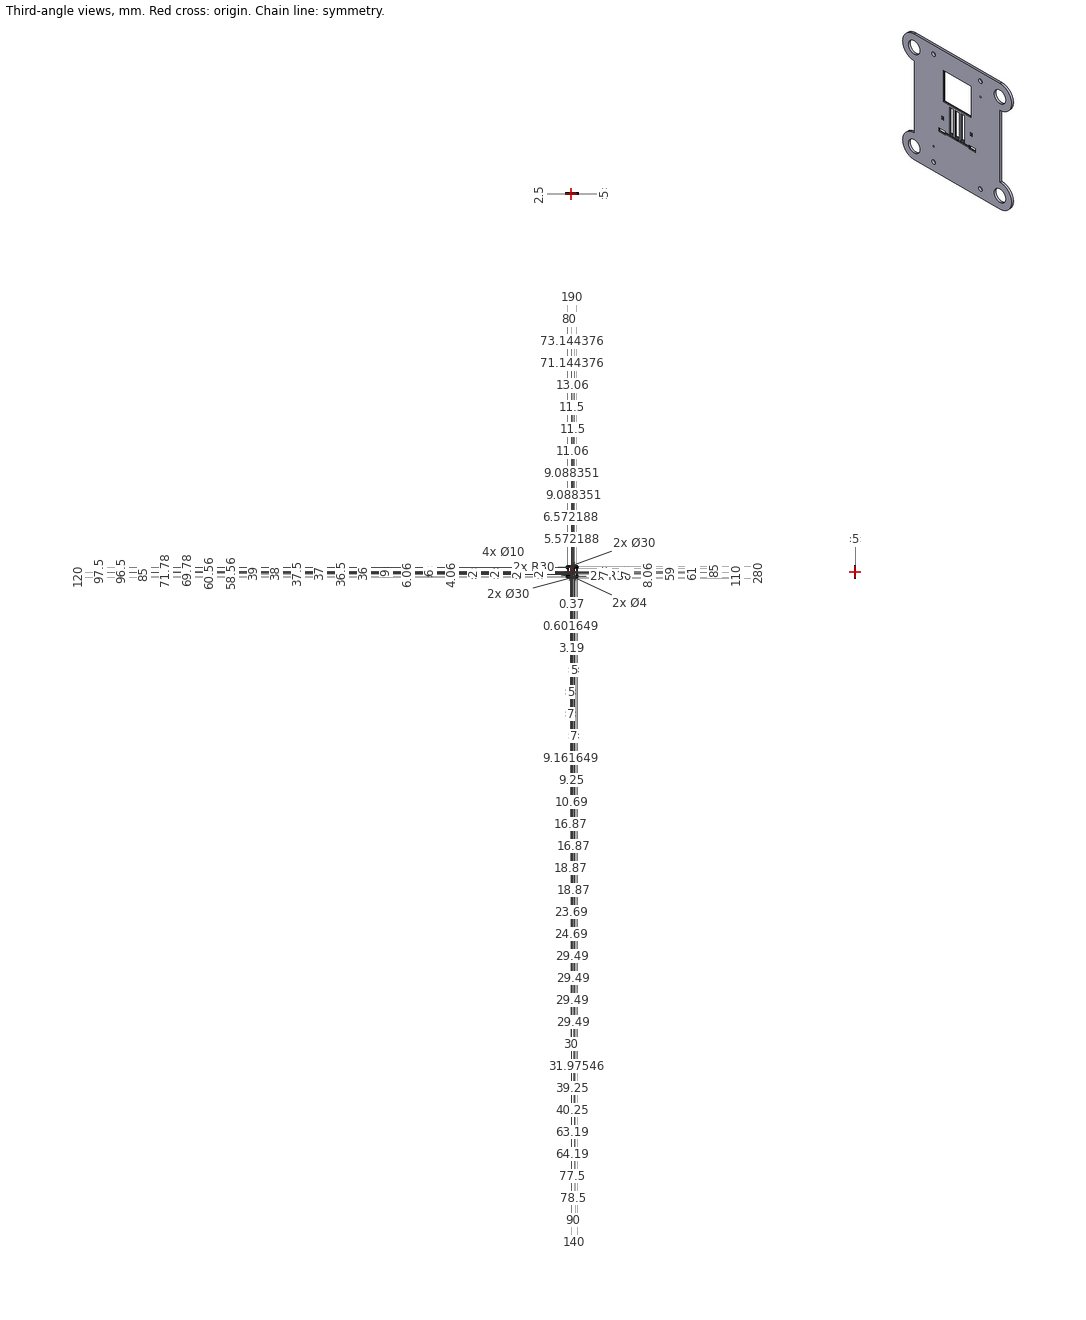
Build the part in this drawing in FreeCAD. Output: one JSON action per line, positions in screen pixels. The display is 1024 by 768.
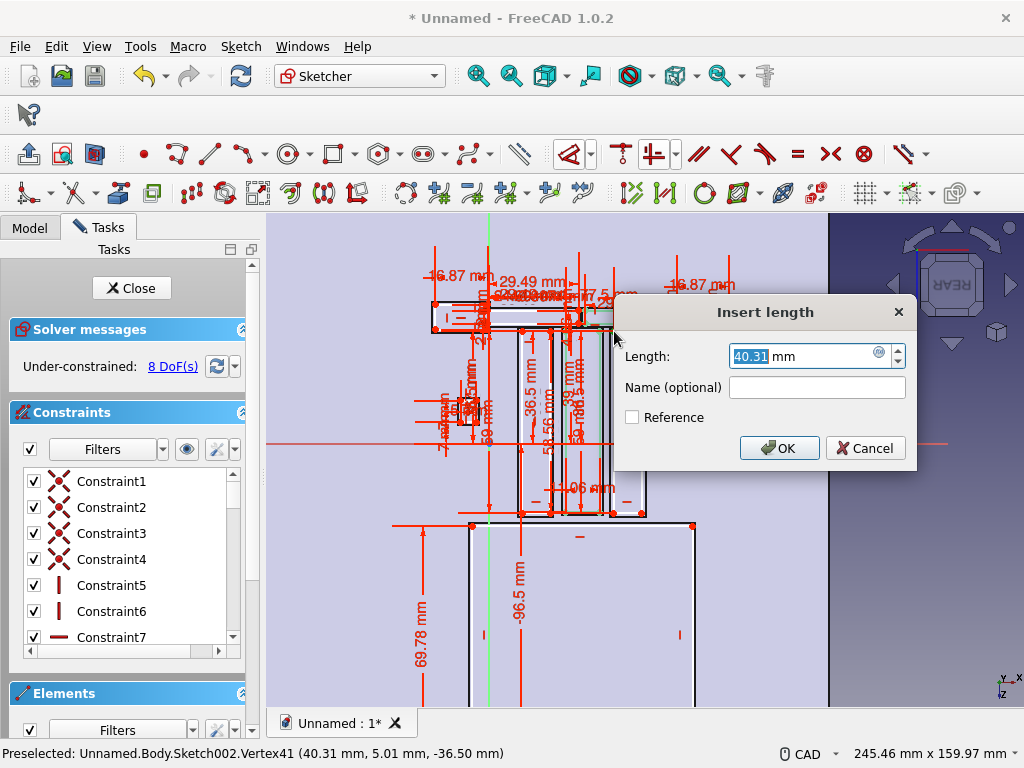
{"action": "type", "text": "40.25"}
{"action": "key", "text": "Return"}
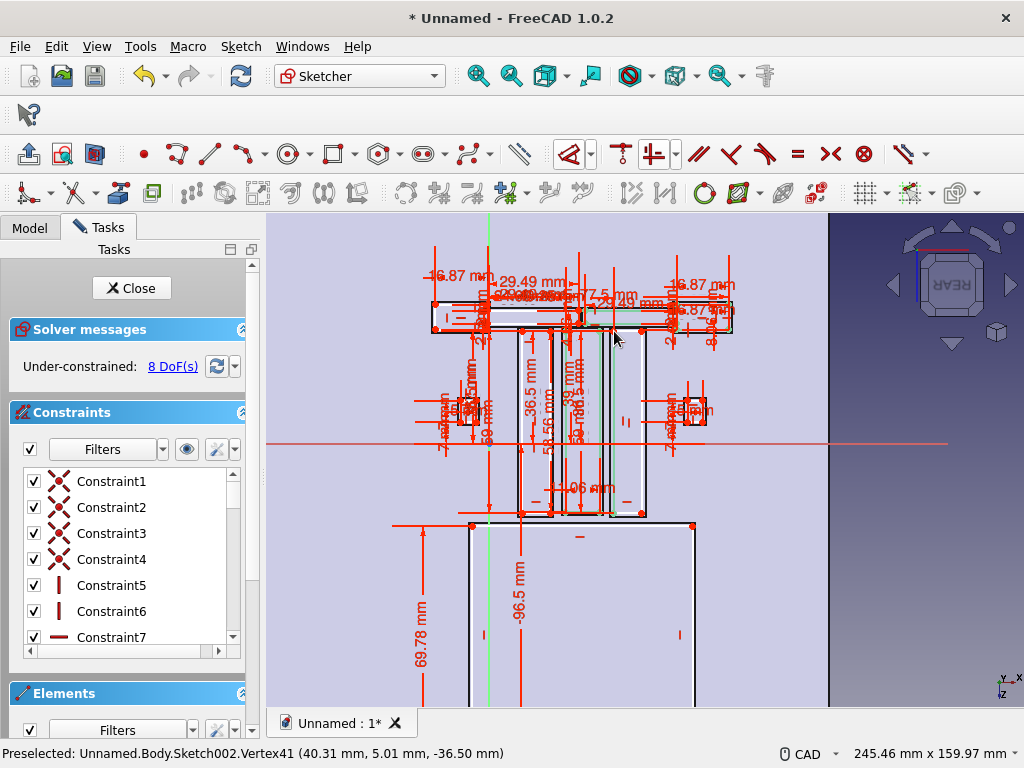
{"action": "left_click", "coordinate": [688, 401]}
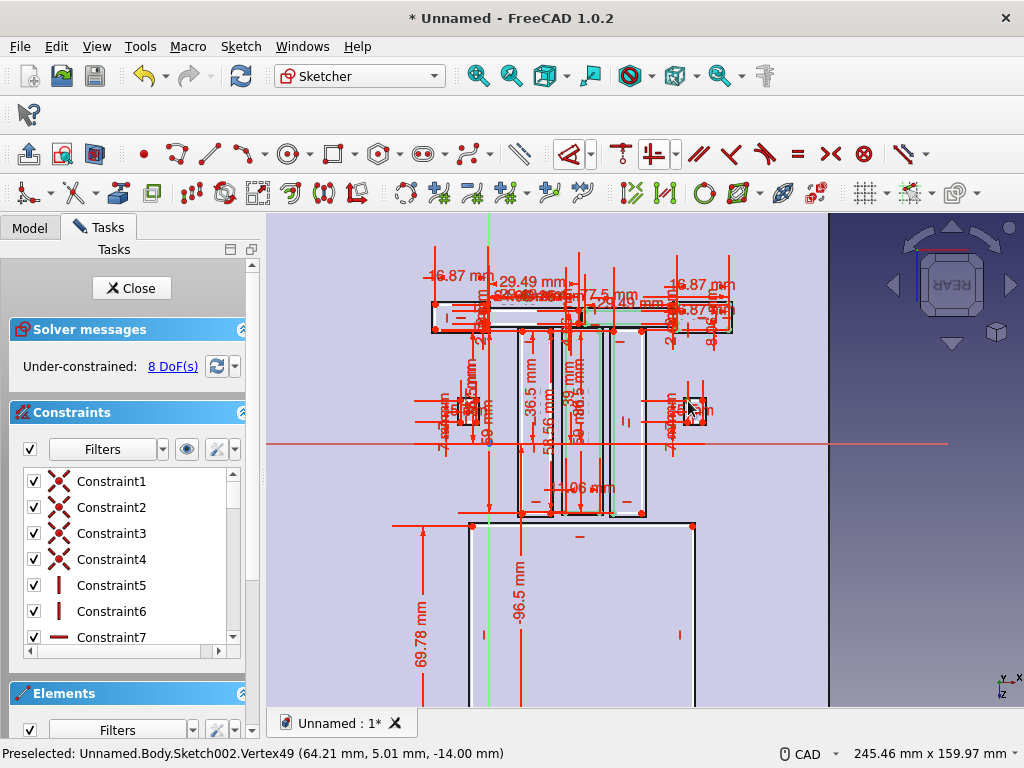
{"action": "key", "text": "l"}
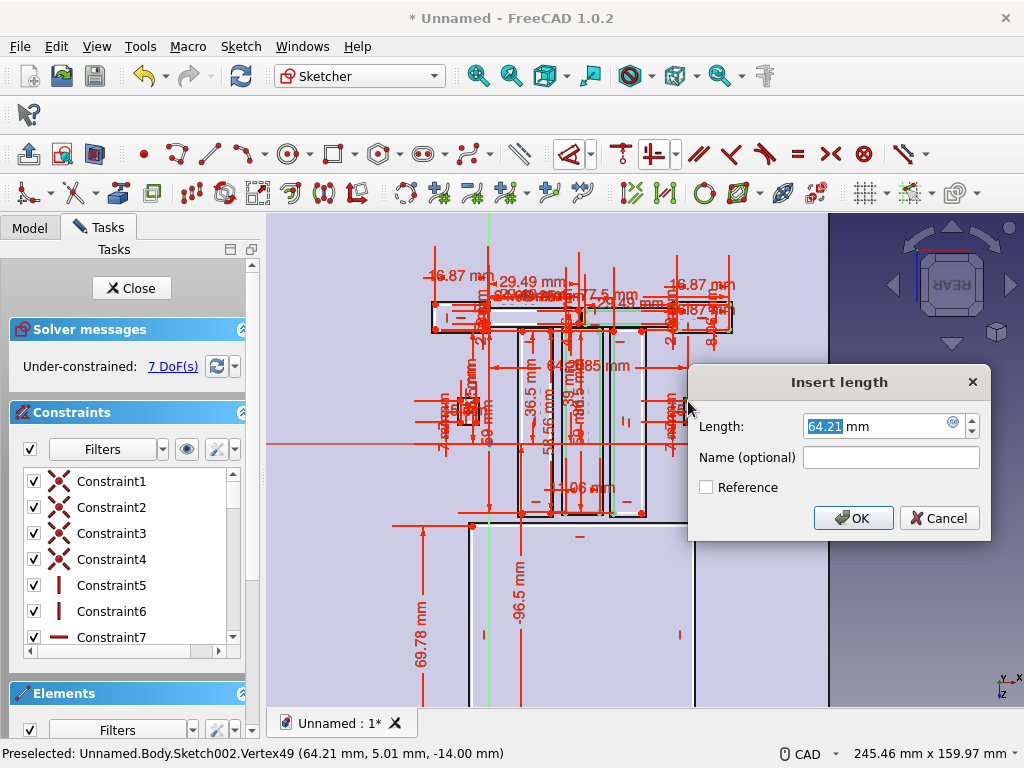
{"action": "type", "text": "64.19"}
{"action": "key", "text": "Return"}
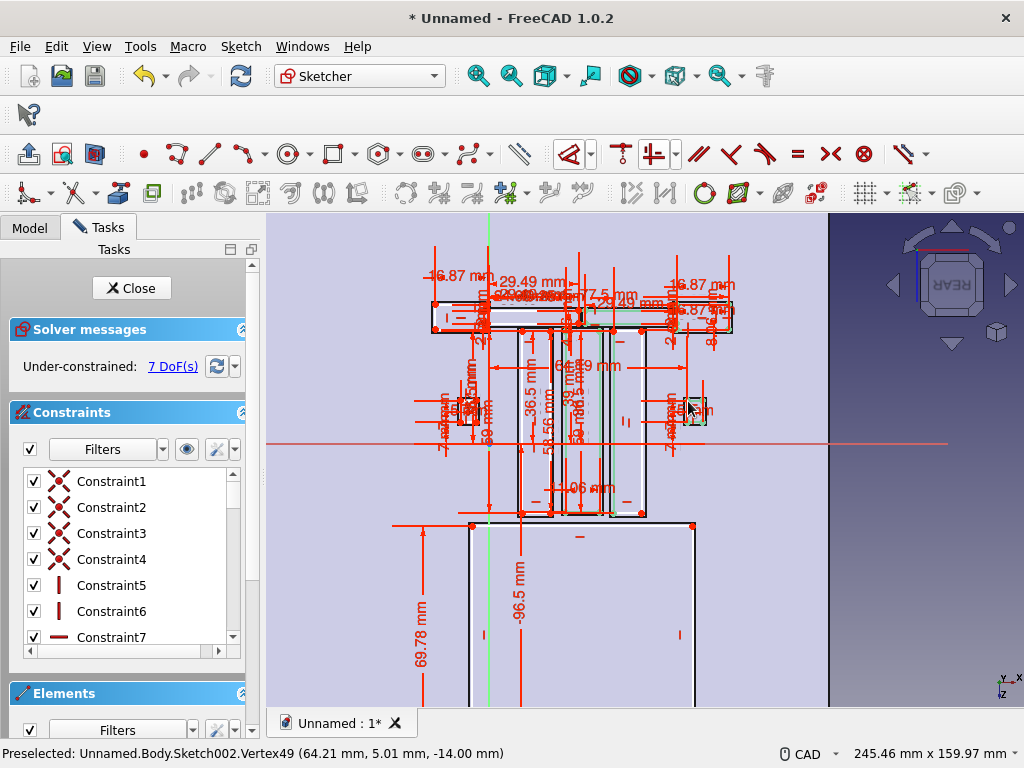
{"action": "left_click", "coordinate": [522, 331]}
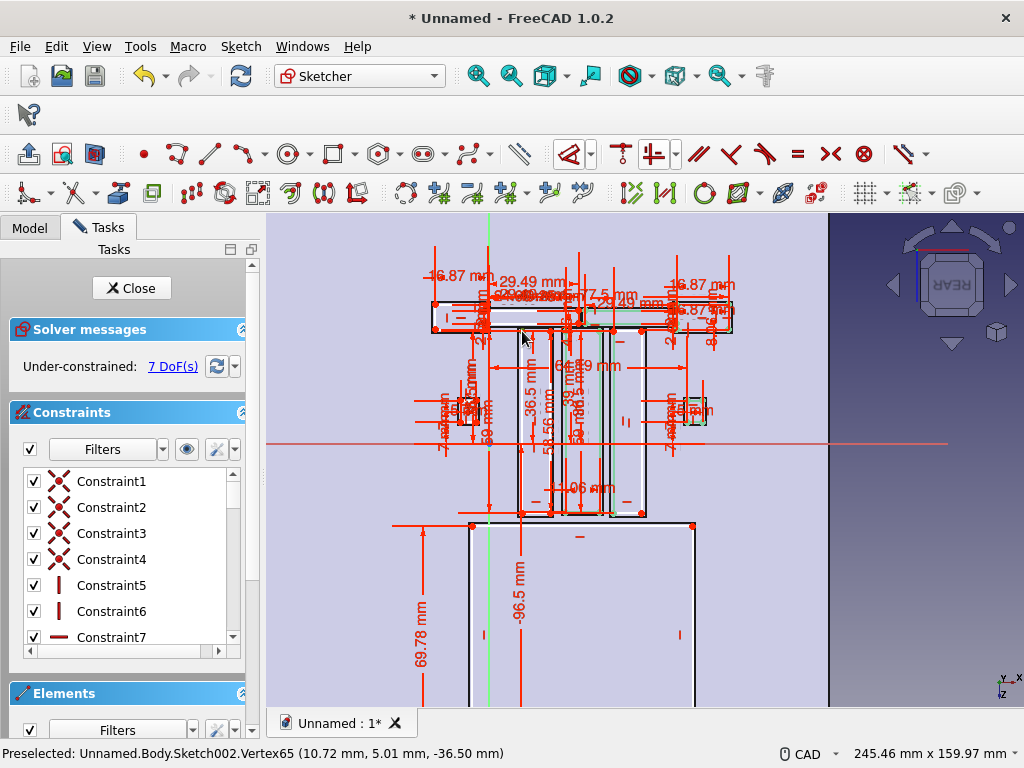
{"action": "key", "text": "l"}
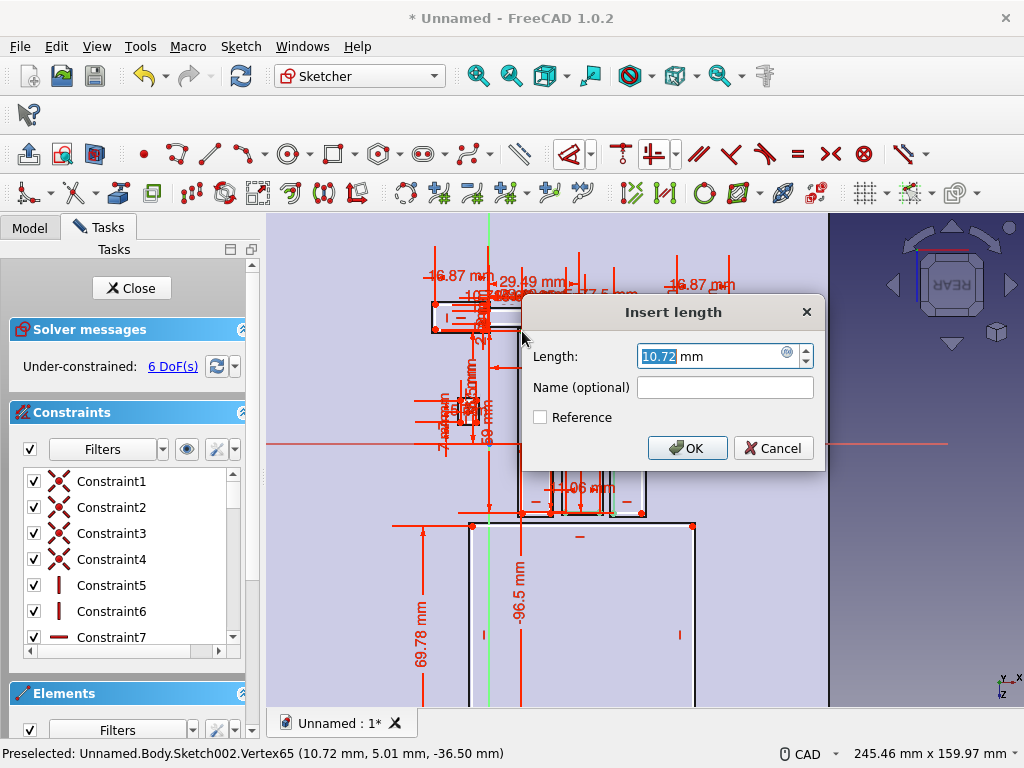
{"action": "type", "text": "10.69"}
{"action": "key", "text": "Return"}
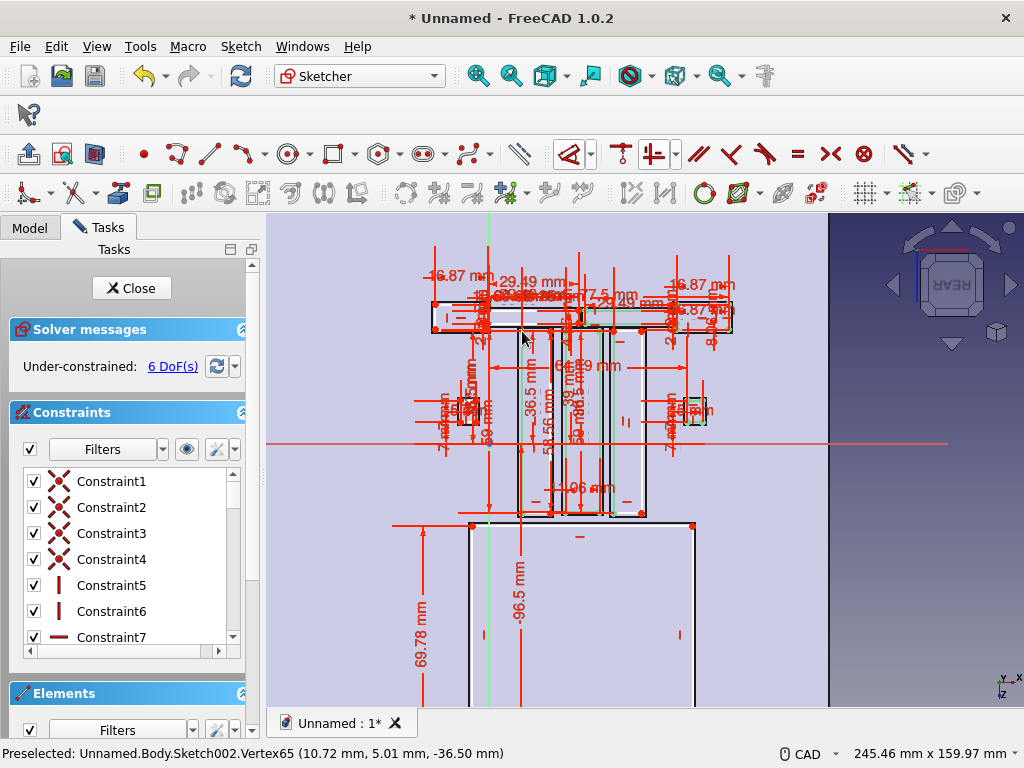
{"action": "scroll", "coordinate": [625, 513], "scroll_direction": "up", "scroll_amount": 2}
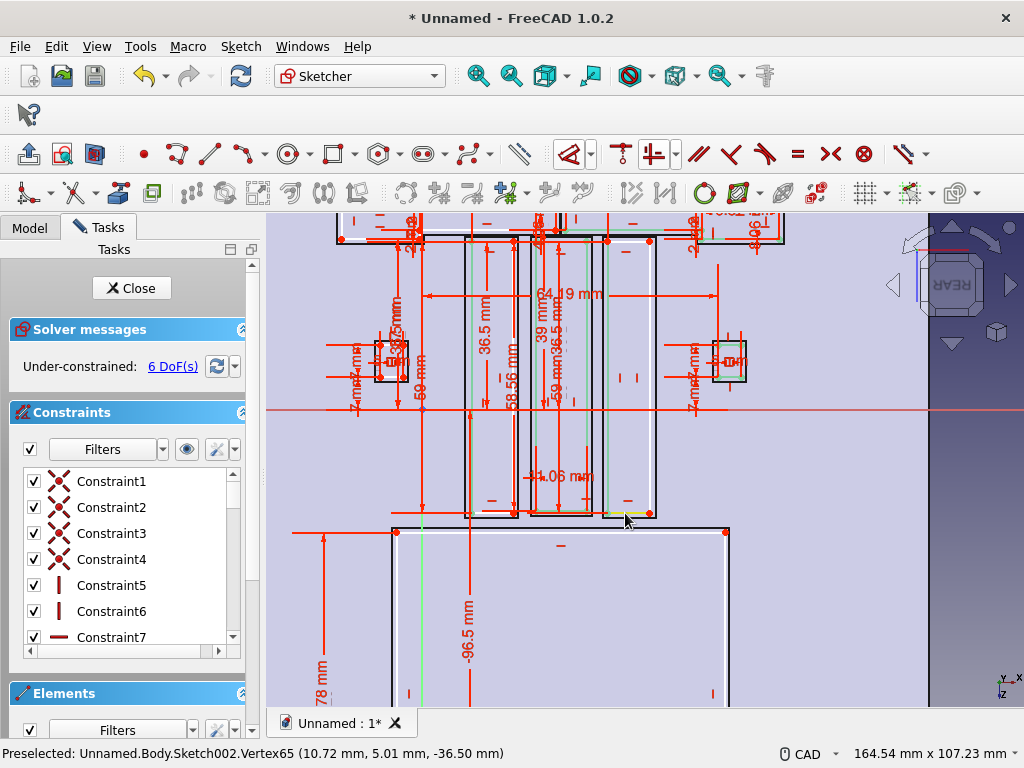
{"action": "left_click", "coordinate": [625, 513]}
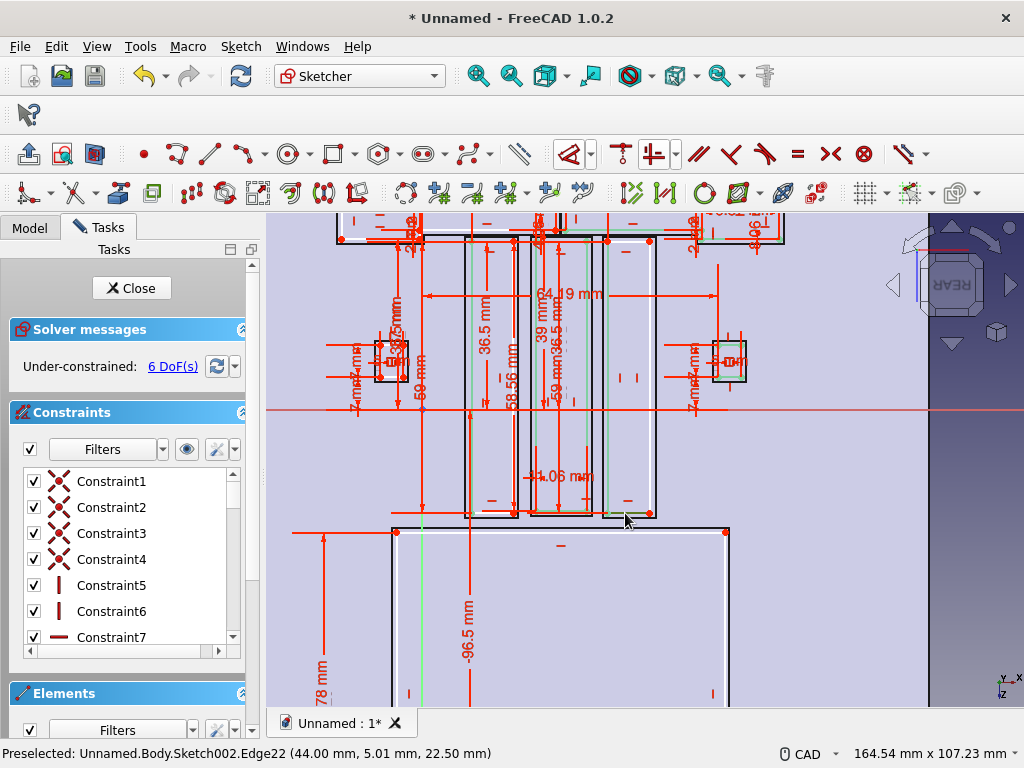
{"action": "key", "text": "l"}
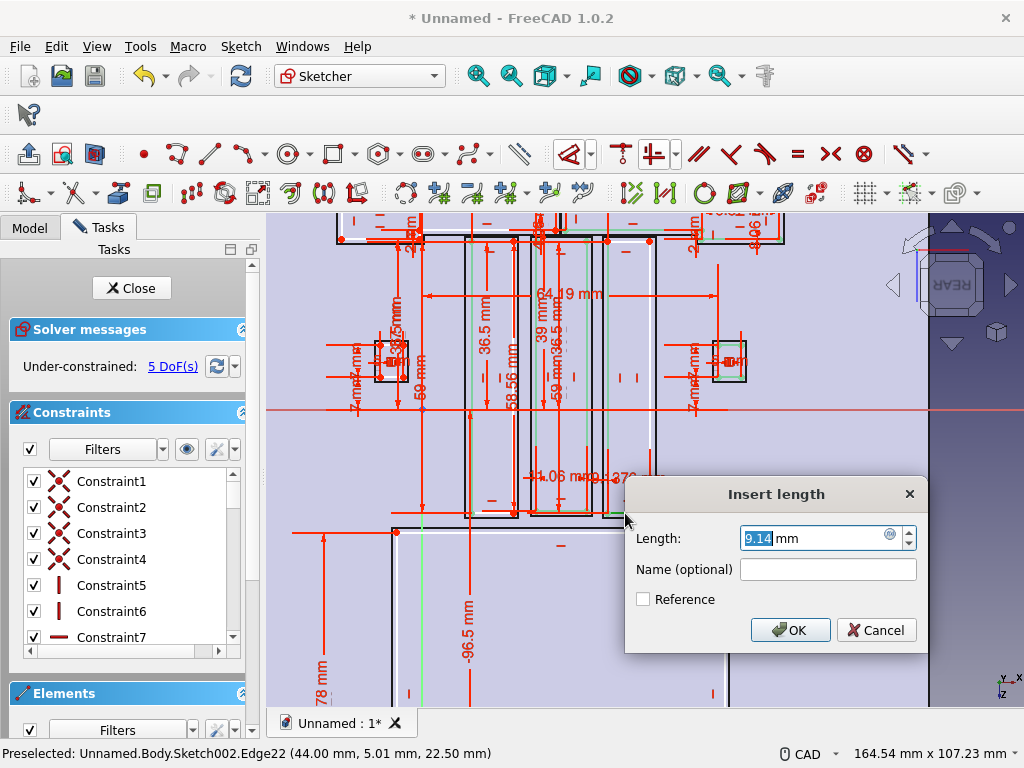
{"action": "type", "text": "9.088351"}
{"action": "key", "text": "Return"}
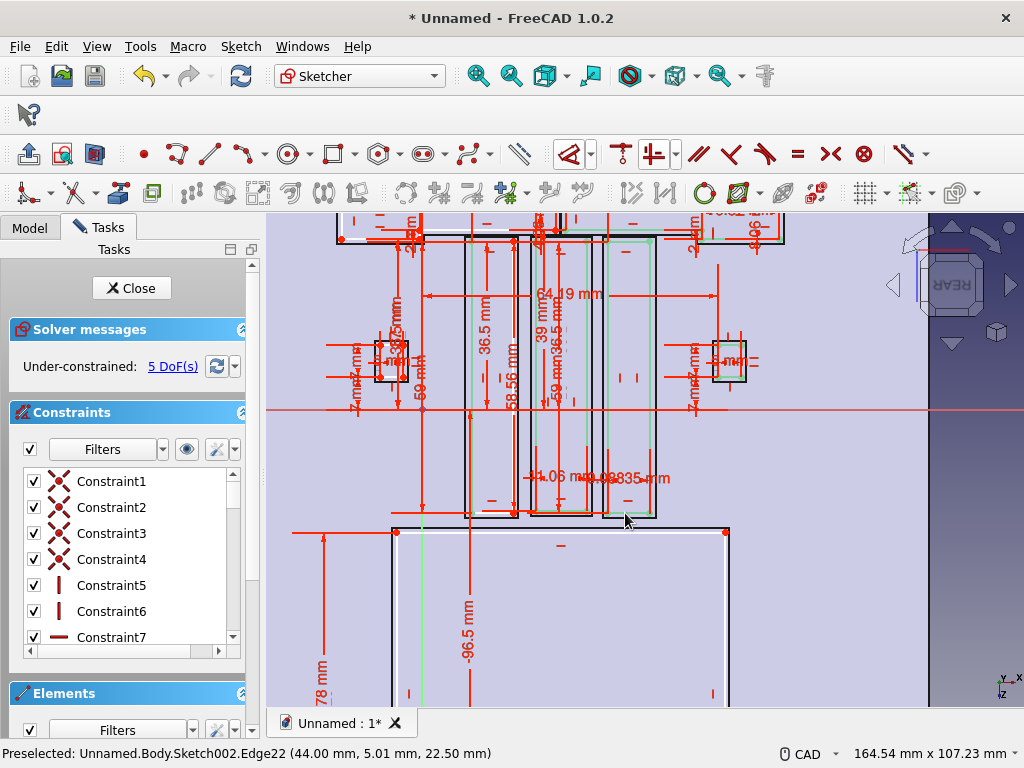
{"action": "left_click", "coordinate": [484, 513]}